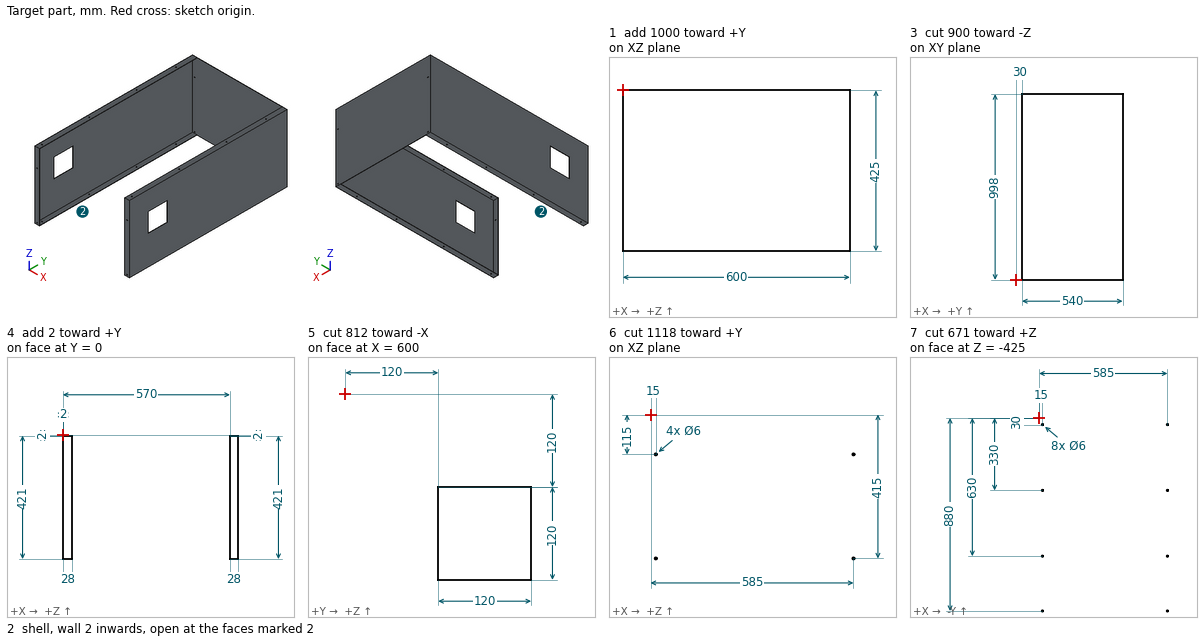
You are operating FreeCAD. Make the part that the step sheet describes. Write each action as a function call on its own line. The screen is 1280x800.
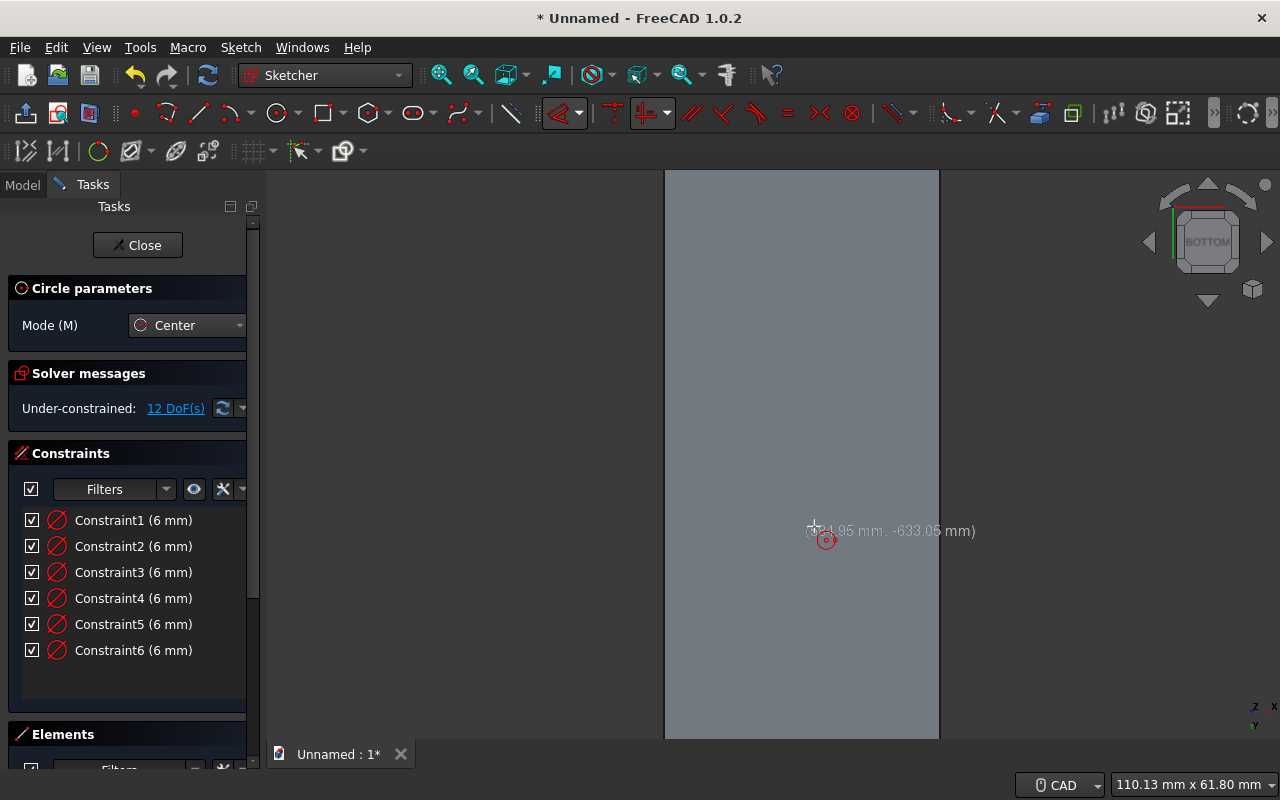
scroll(840, 543, down, 15)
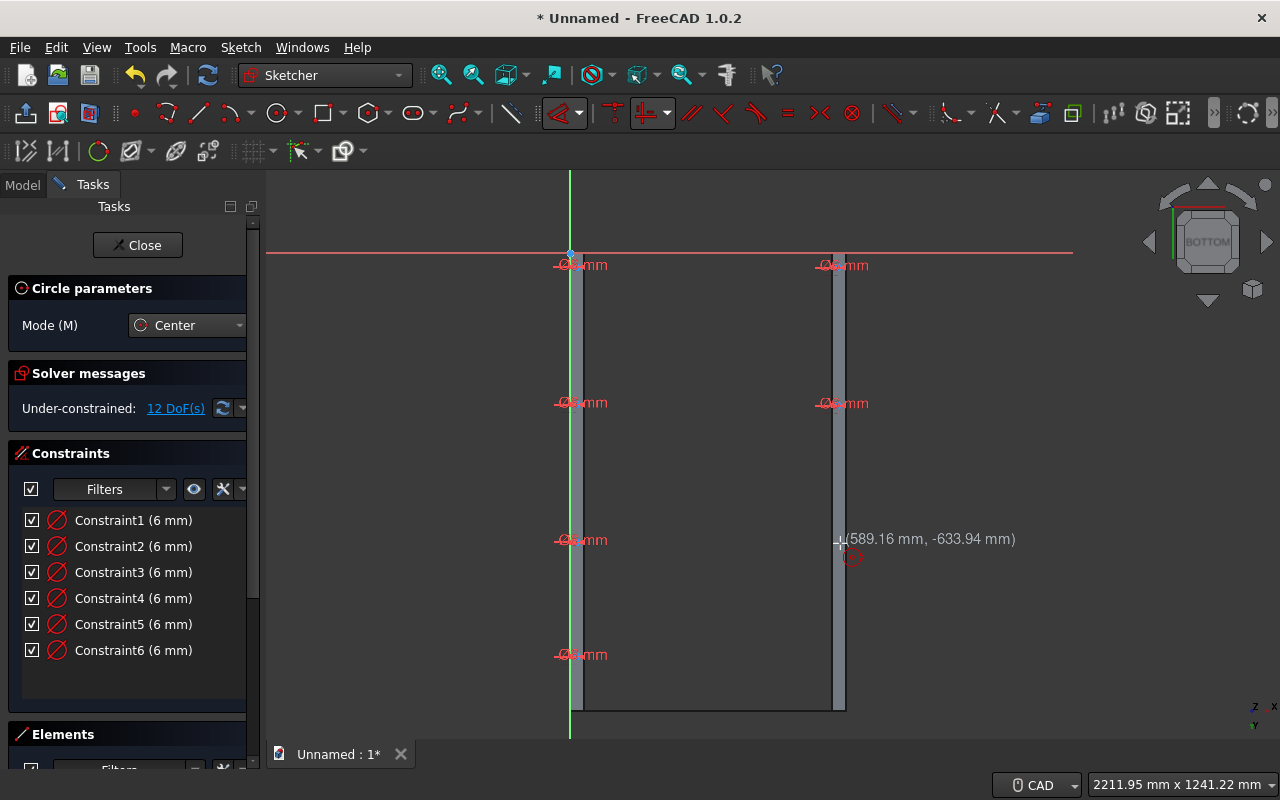
click(839, 542)
move(840, 541)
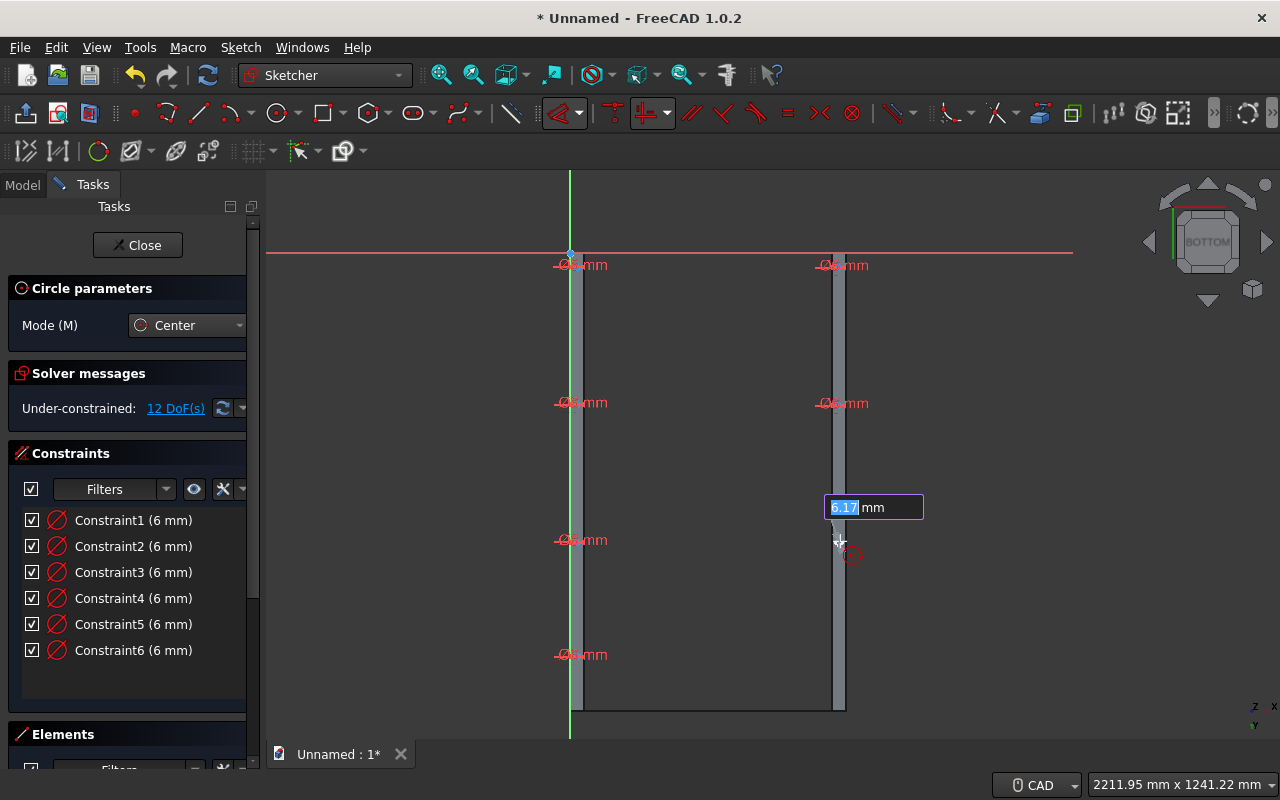
text(6)
key(Return)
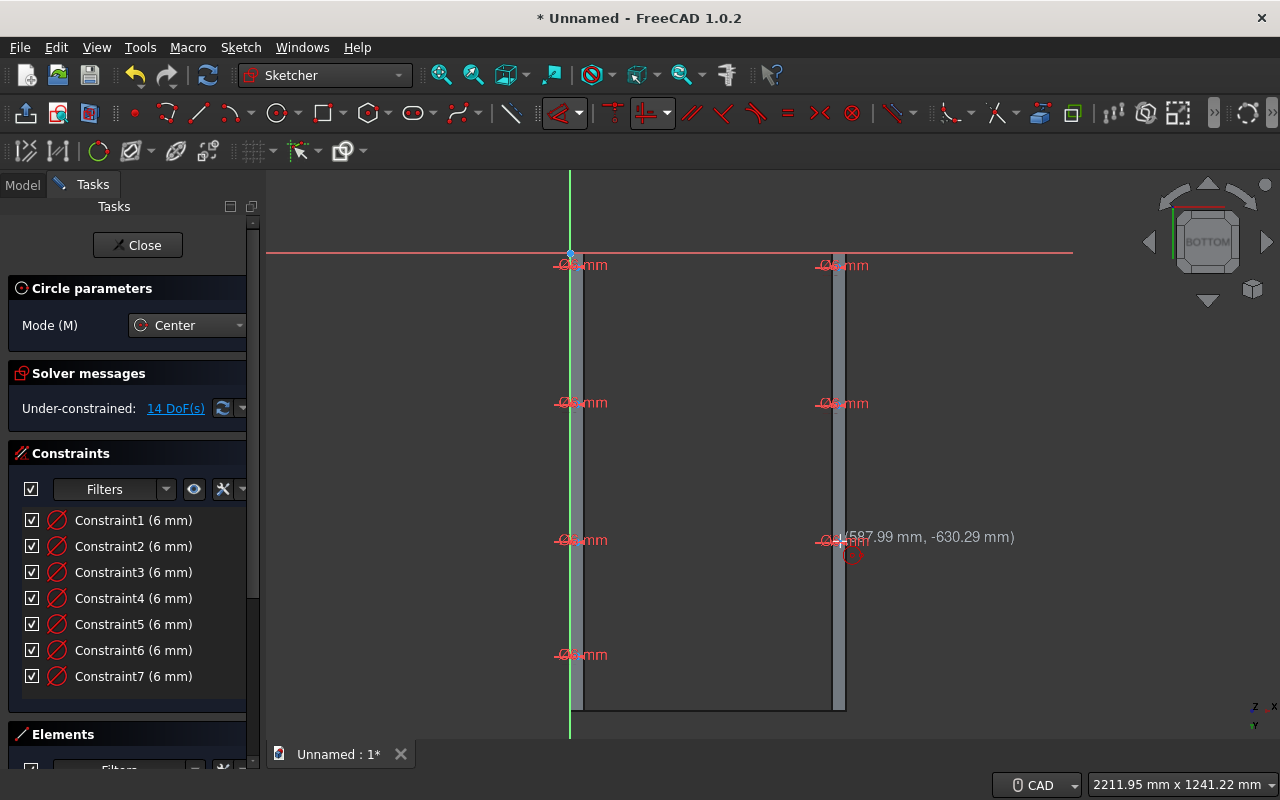
scroll(839, 656, up, 15)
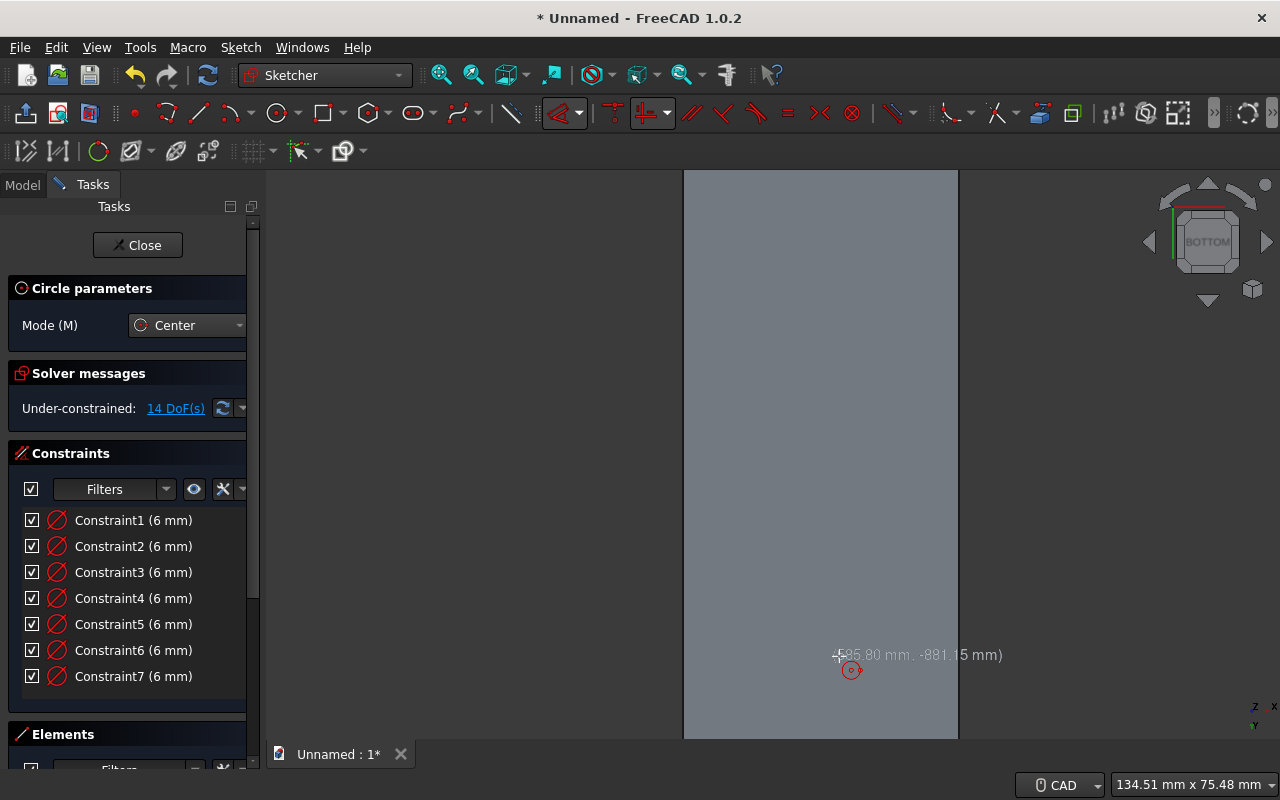
scroll(839, 656, down, 15)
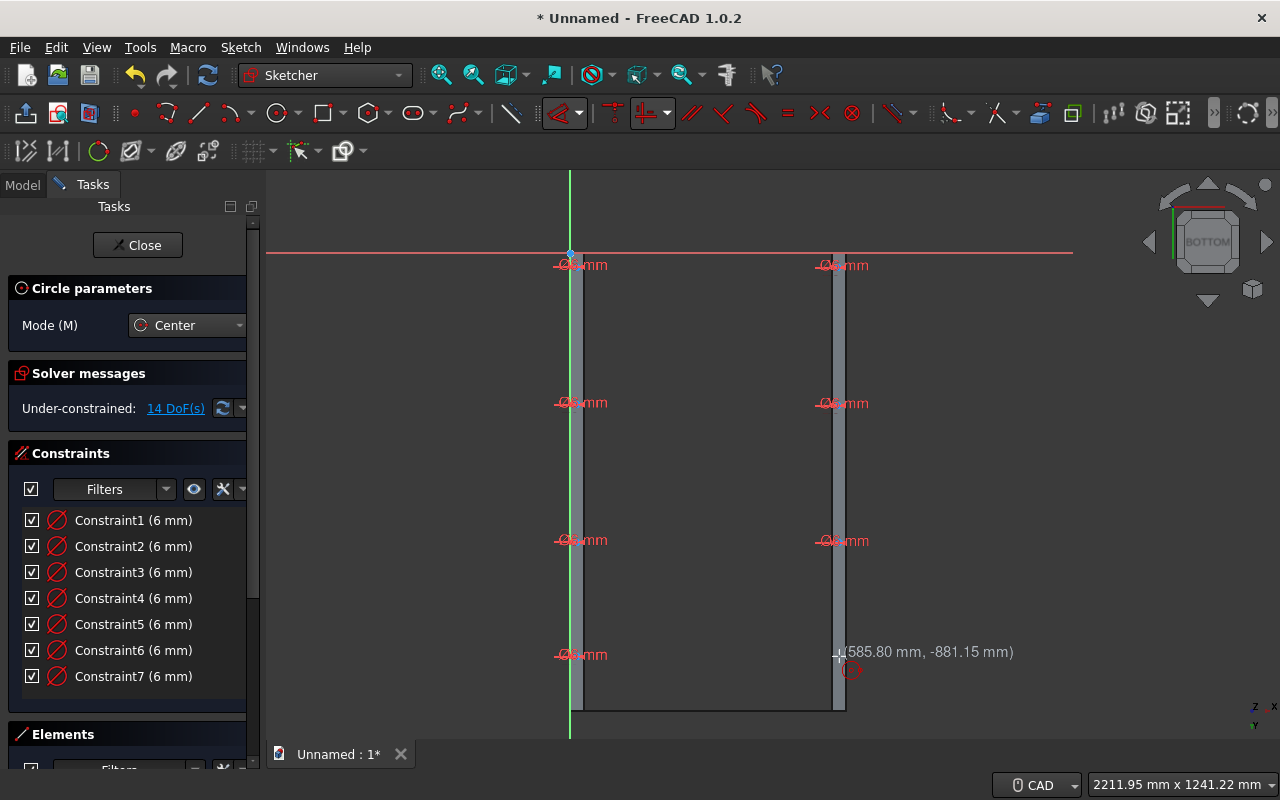
click(839, 656)
move(840, 655)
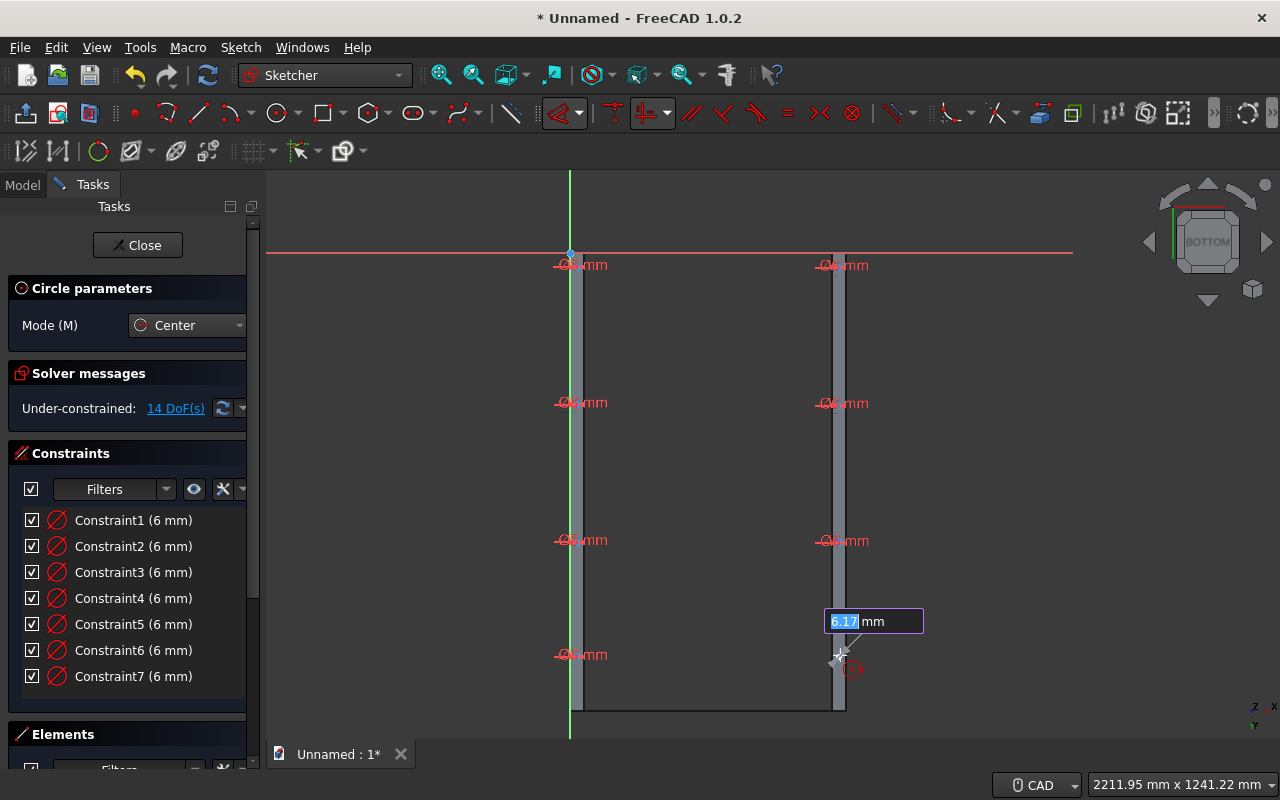
text(6)
key(Return)
key(Escape)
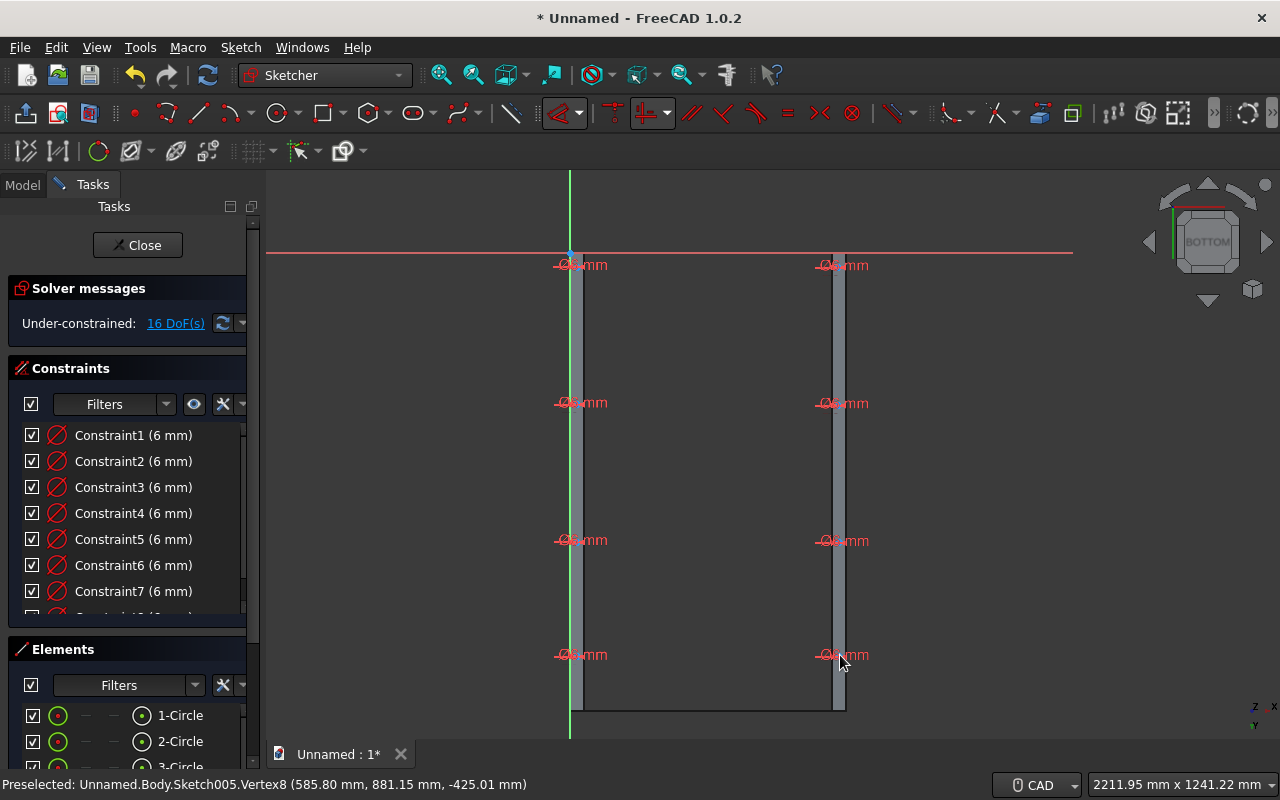
click(577, 267)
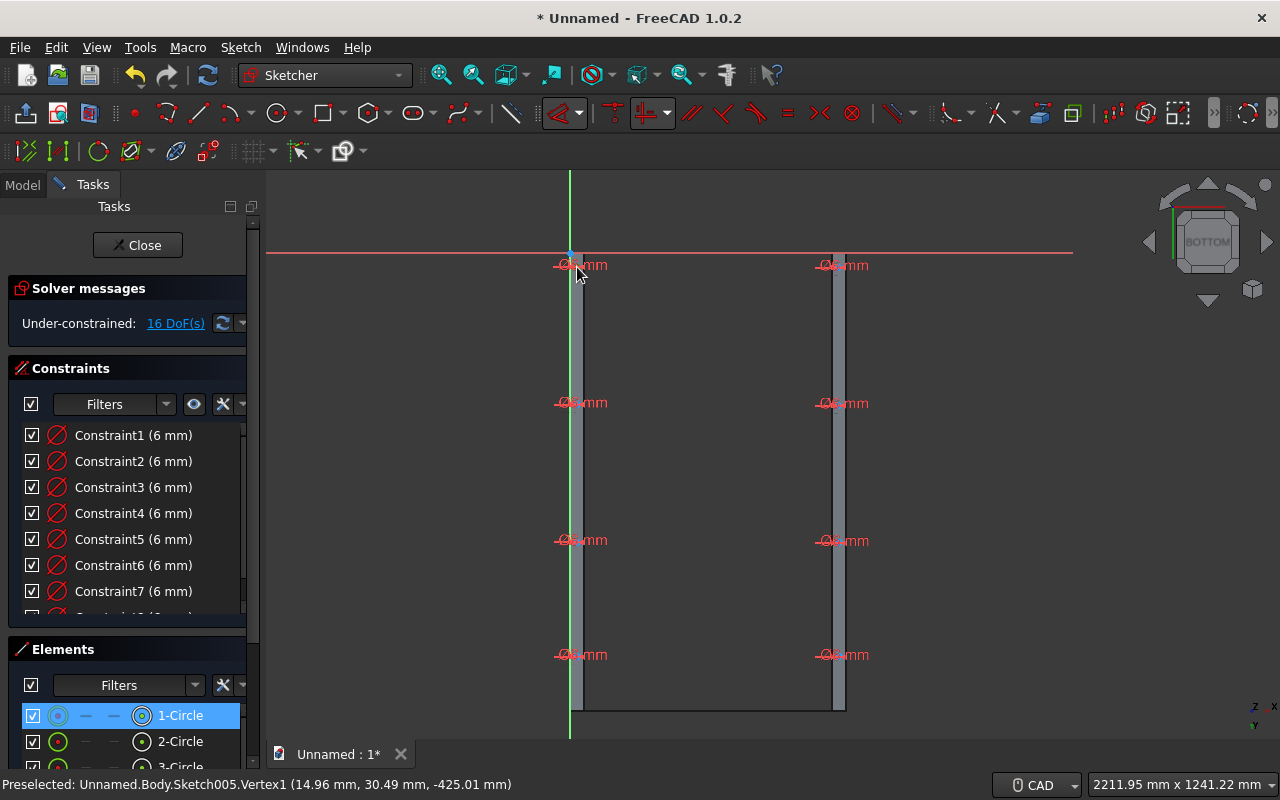
click(577, 405)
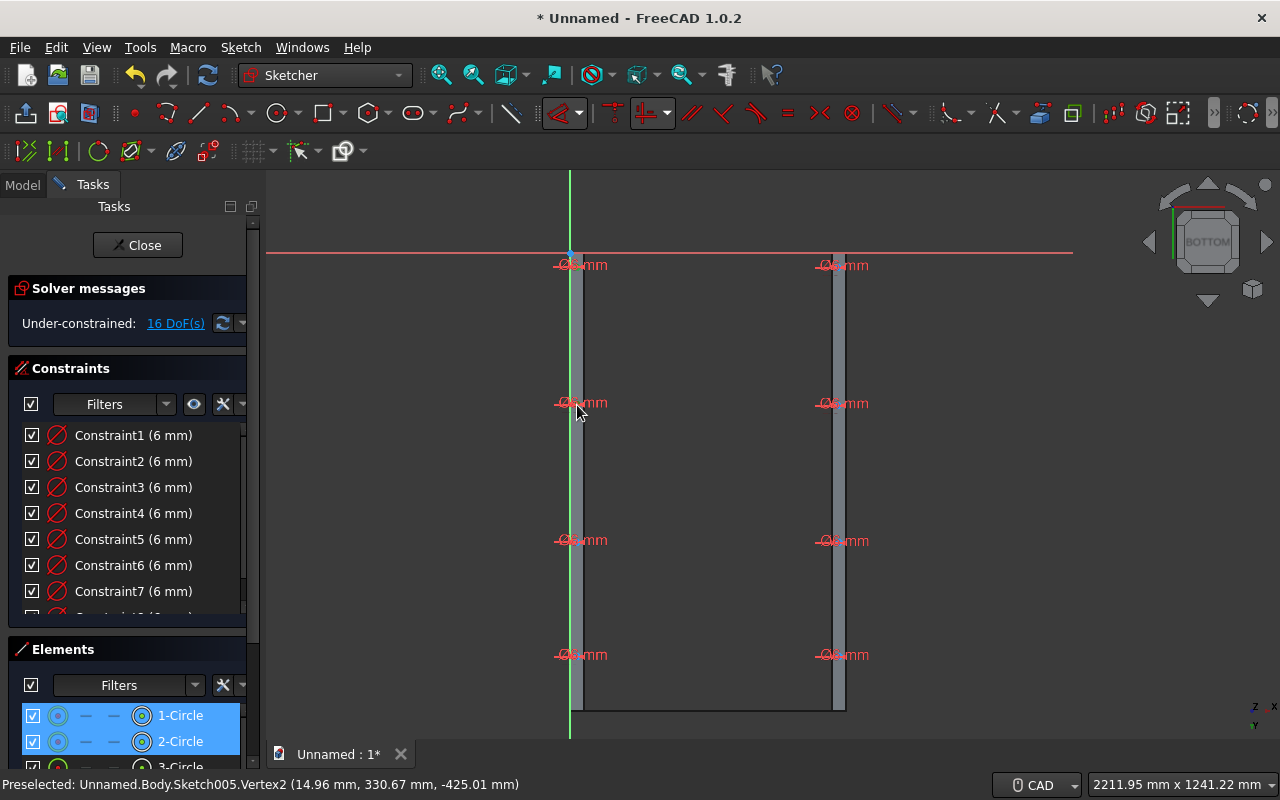
click(670, 114)